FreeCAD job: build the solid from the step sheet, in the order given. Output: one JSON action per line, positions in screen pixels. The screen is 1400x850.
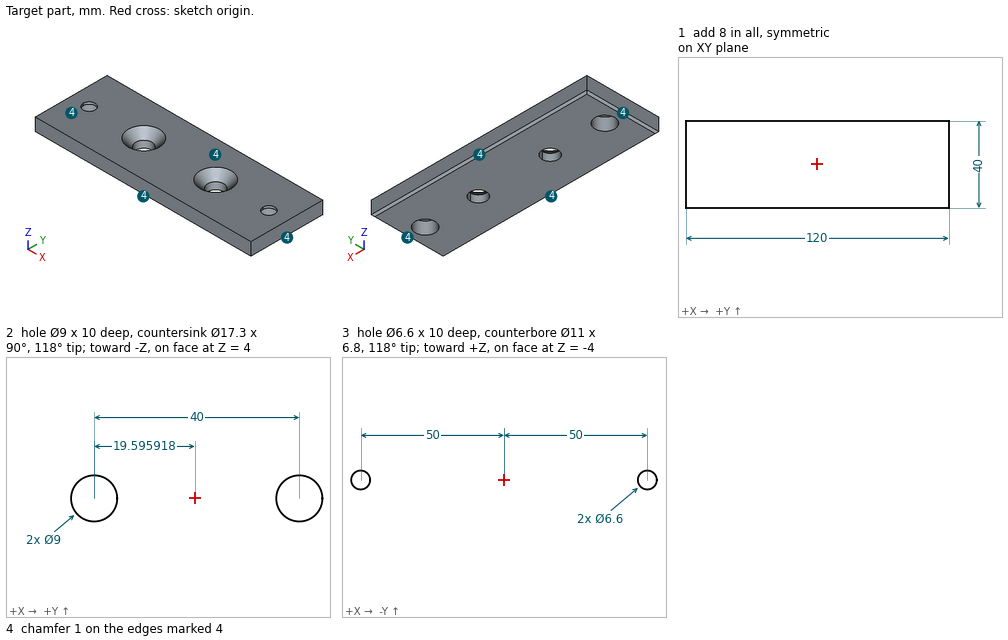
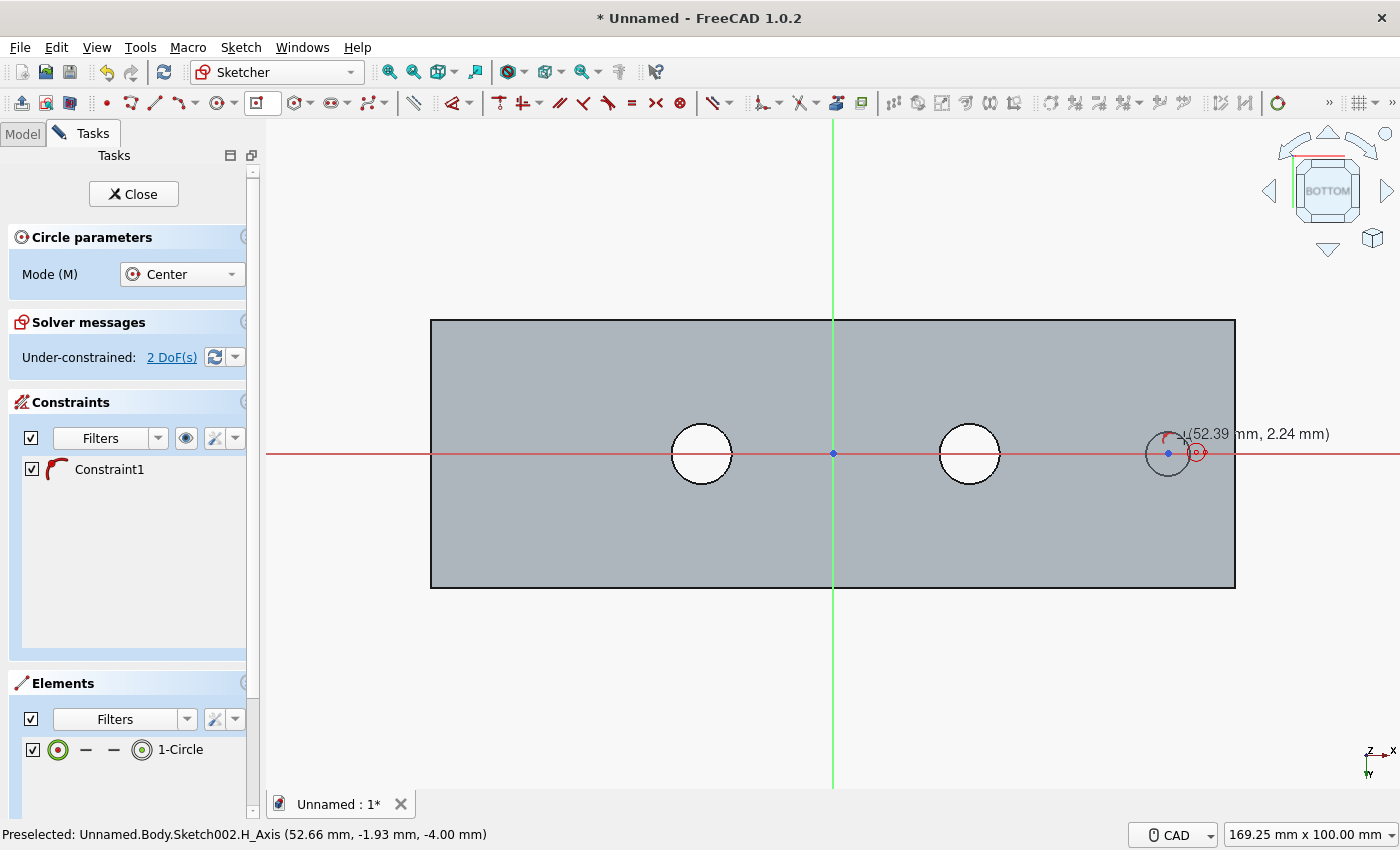
{"action": "left_click", "coordinate": [498, 454]}
{"action": "left_click", "coordinate": [514, 438]}
{"action": "key", "text": "Escape"}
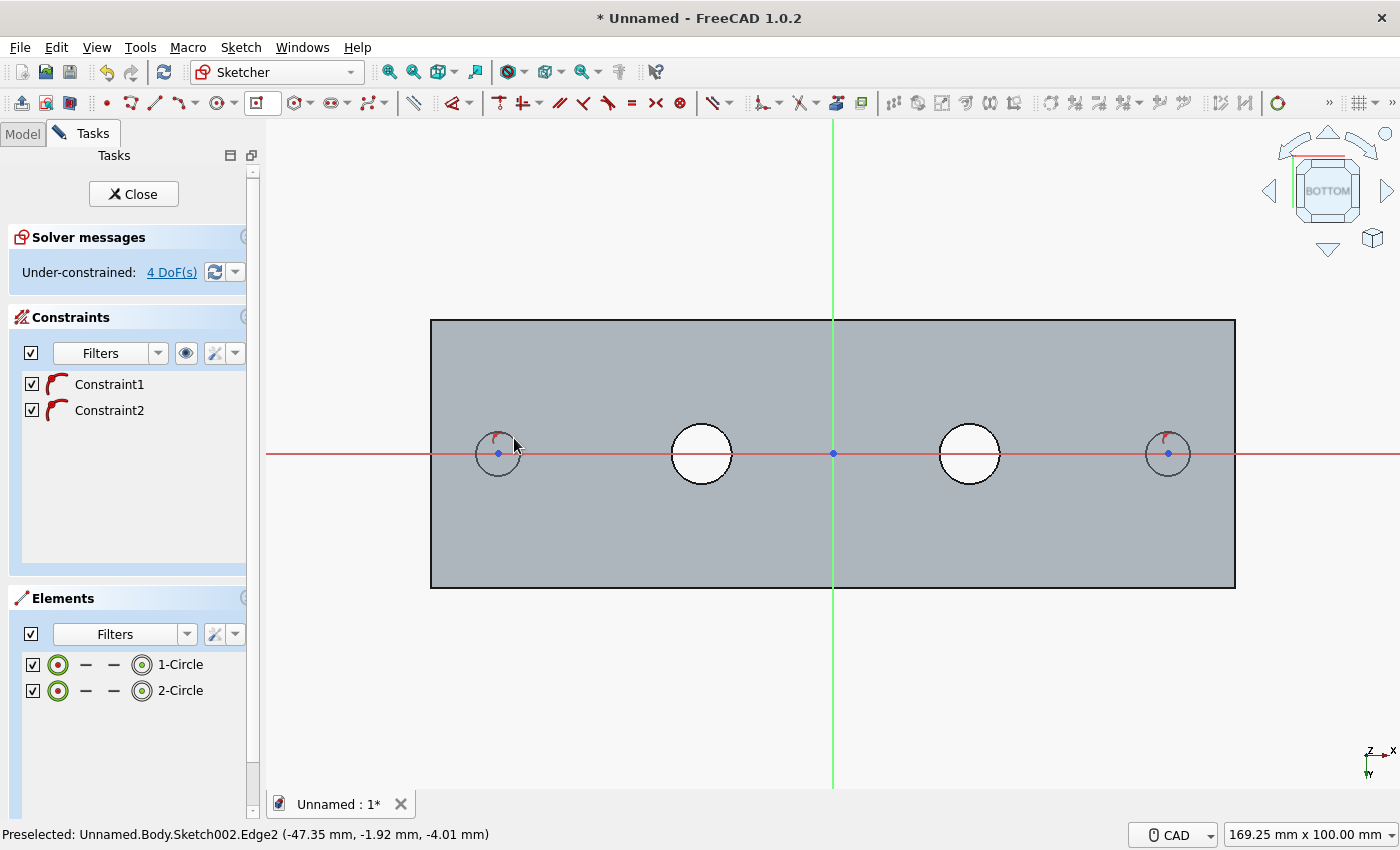
{"action": "left_click", "coordinate": [1183, 438]}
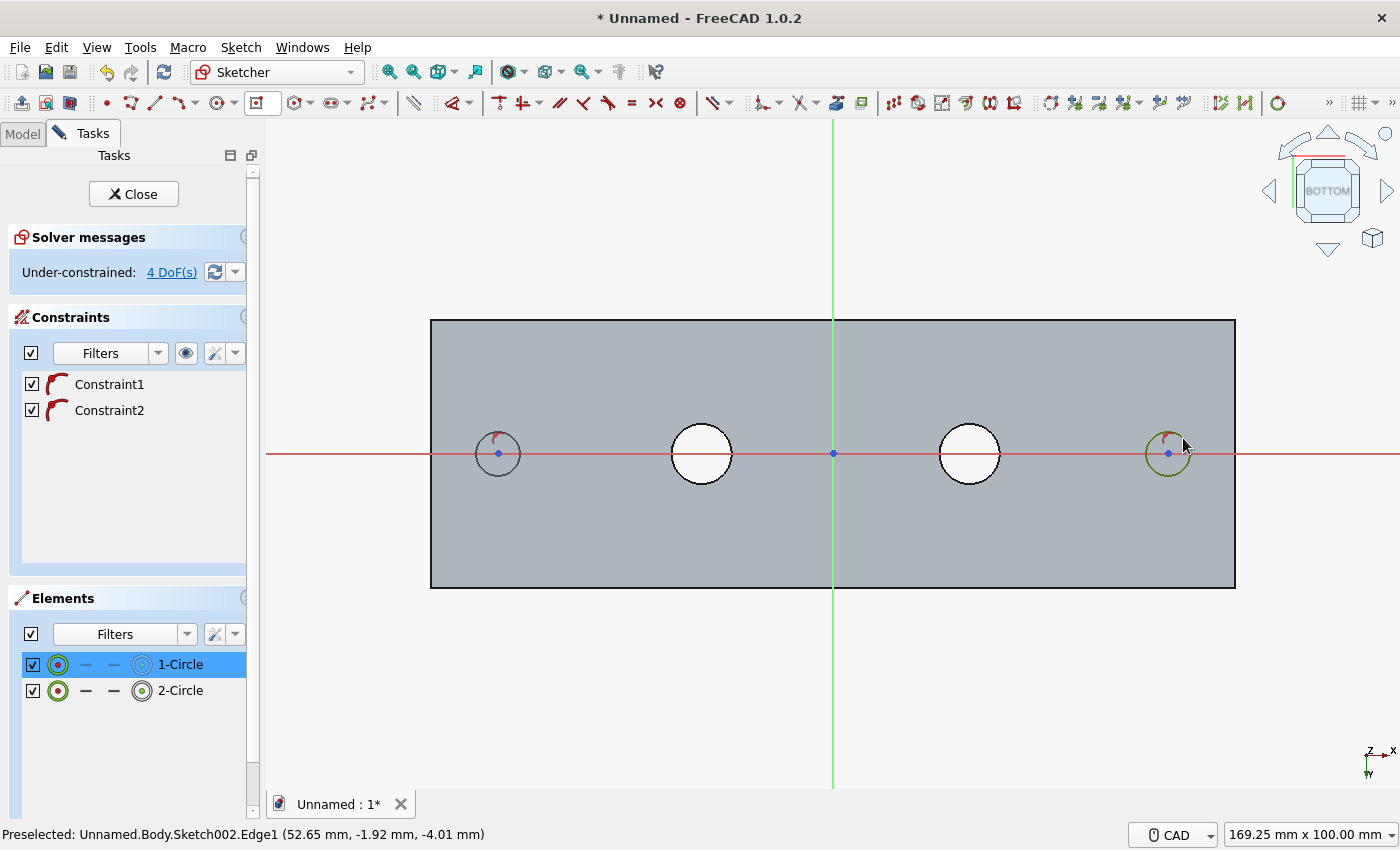
{"action": "left_click", "coordinate": [513, 438]}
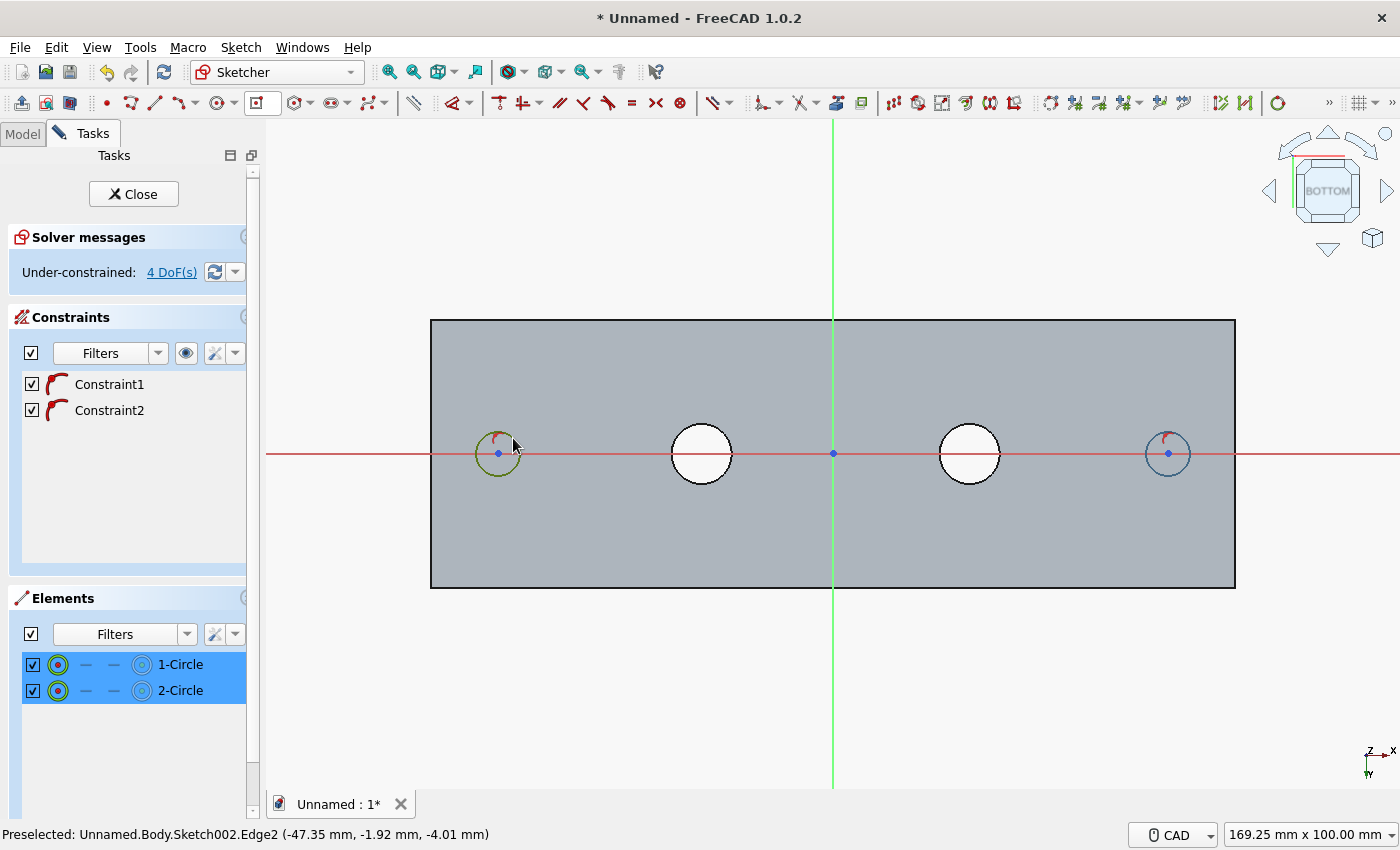
{"action": "left_click", "coordinate": [632, 104]}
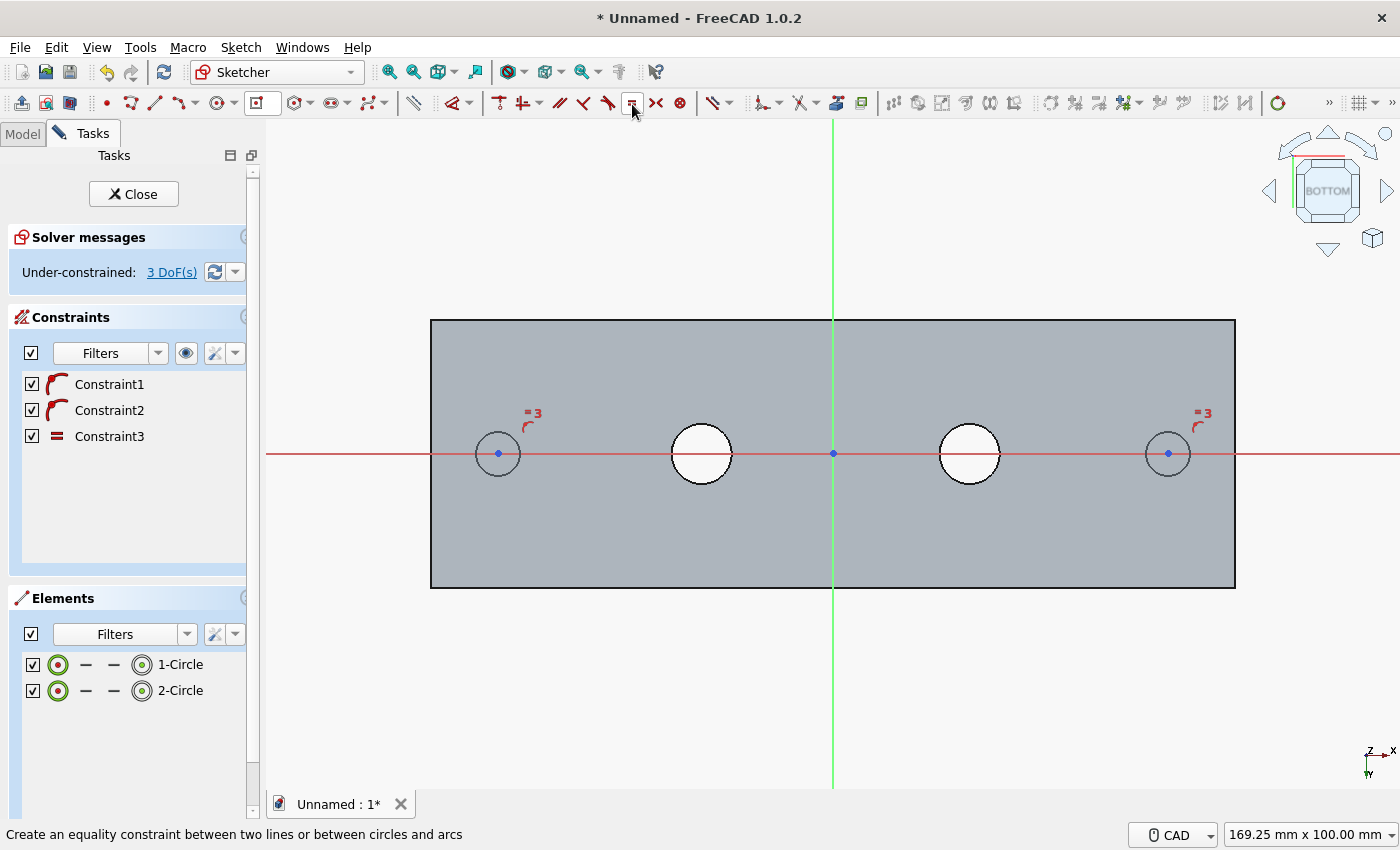
{"action": "left_click", "coordinate": [1183, 438]}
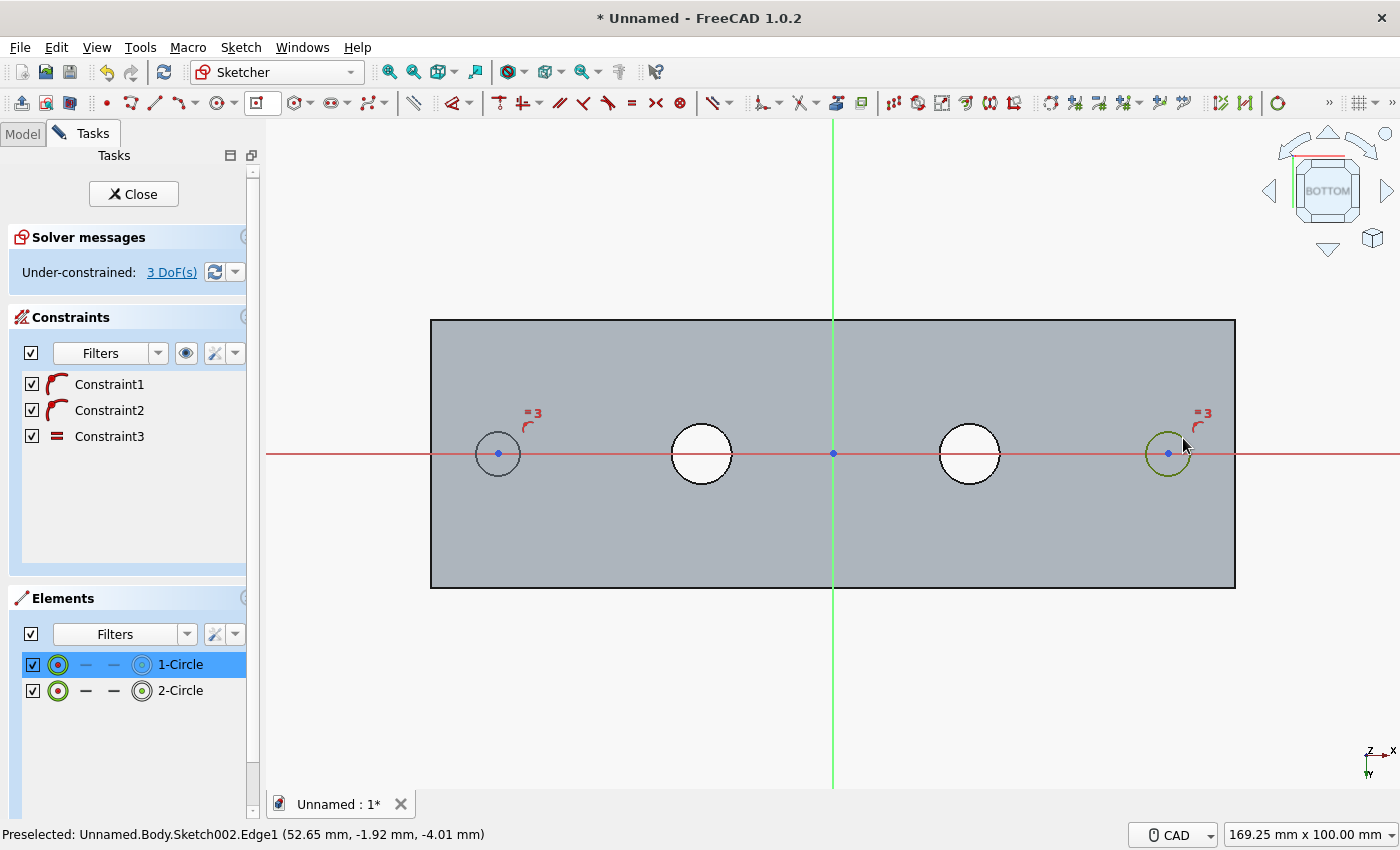
{"action": "key", "text": "k o"}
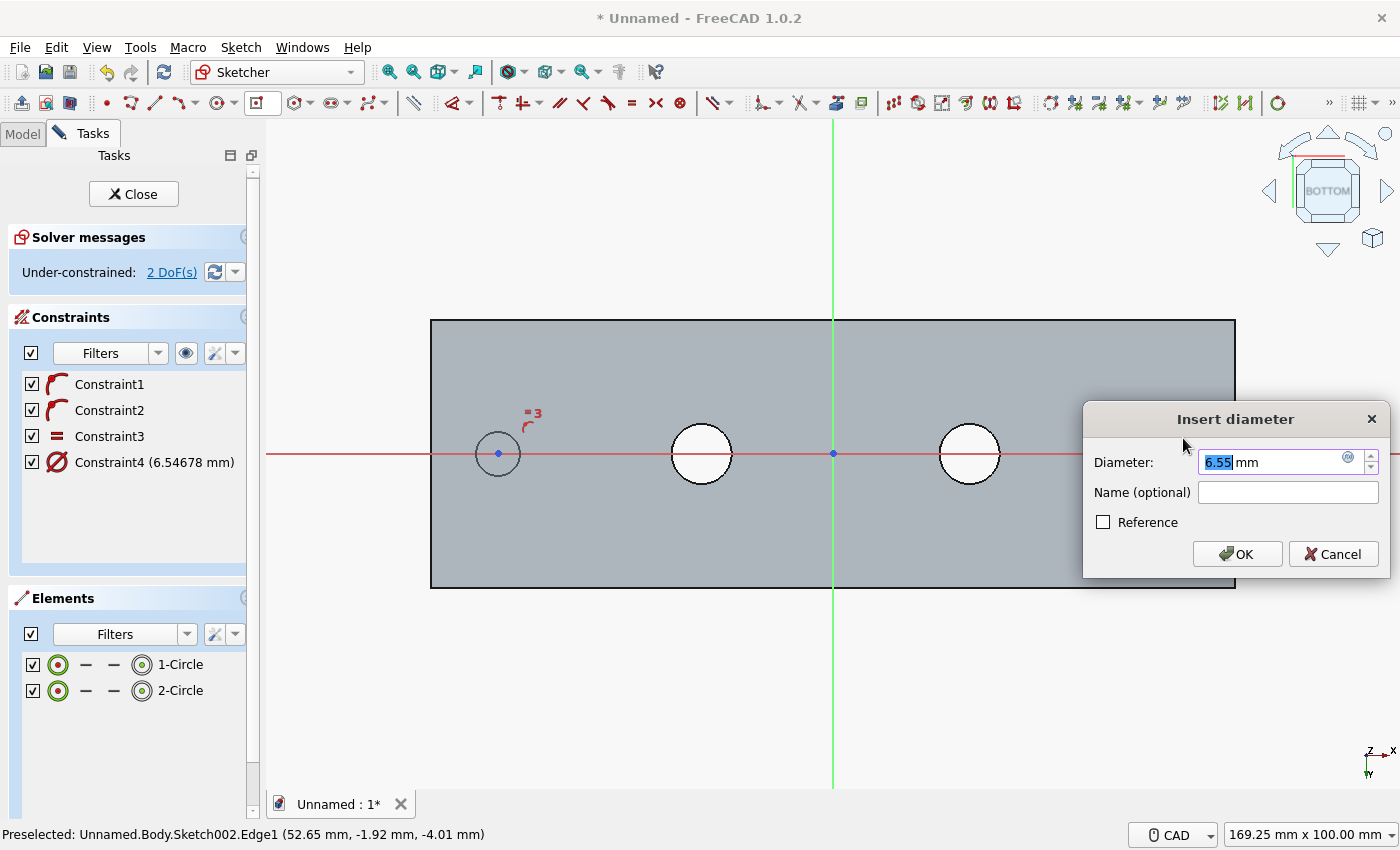
{"action": "type", "text": "6.6"}
{"action": "key", "text": "Return"}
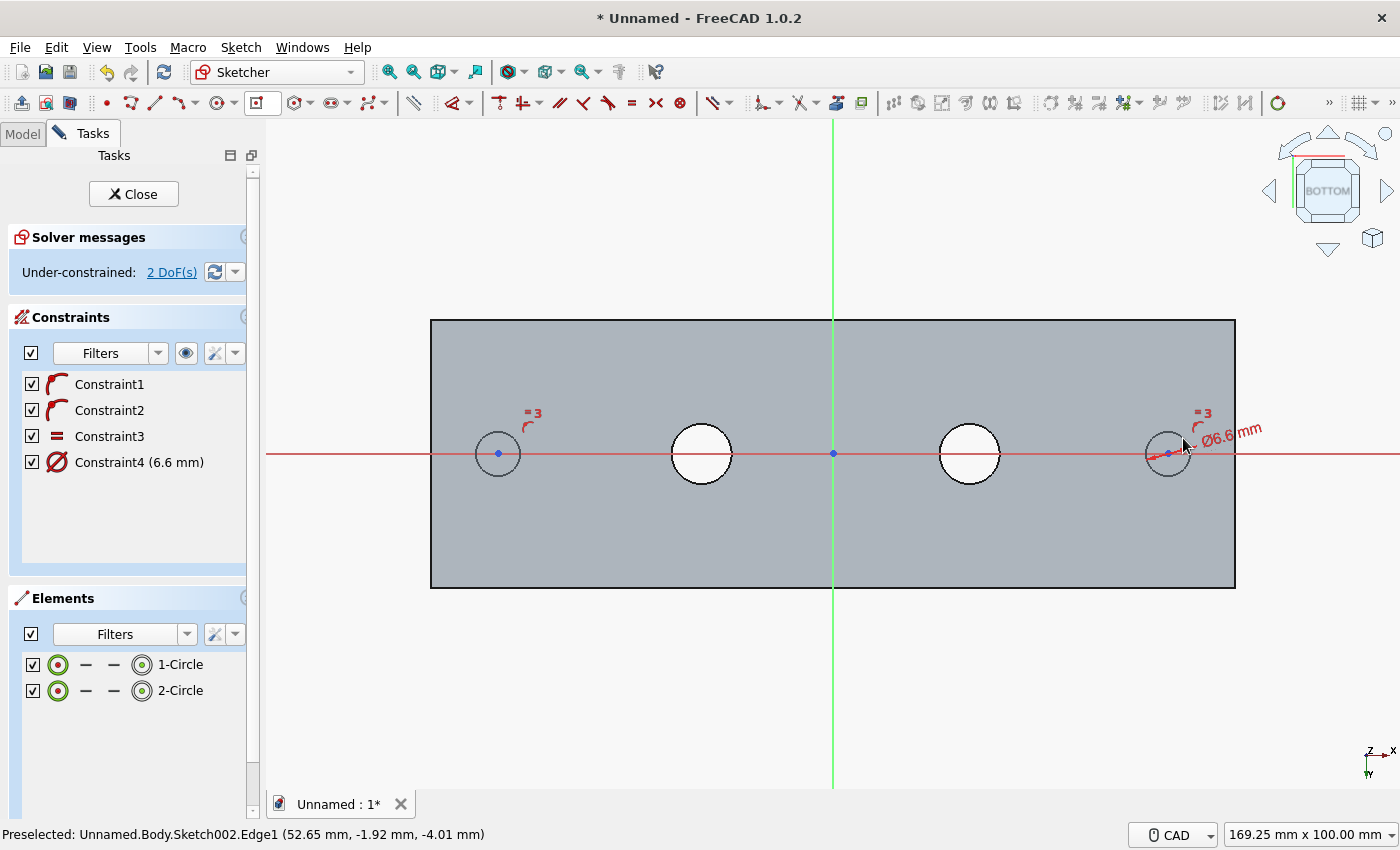
{"action": "left_click", "coordinate": [1168, 454]}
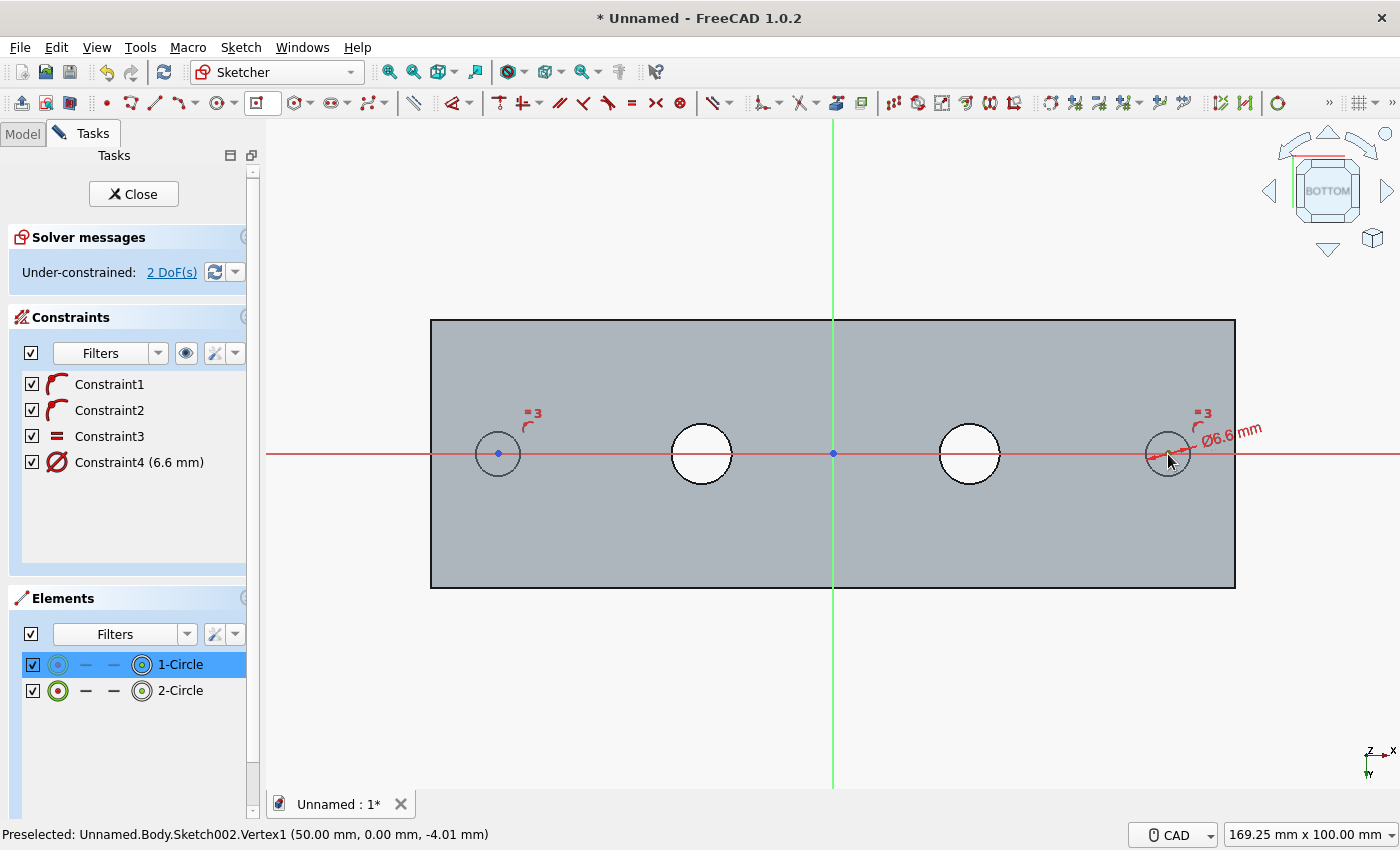
{"action": "left_click", "coordinate": [472, 104]}